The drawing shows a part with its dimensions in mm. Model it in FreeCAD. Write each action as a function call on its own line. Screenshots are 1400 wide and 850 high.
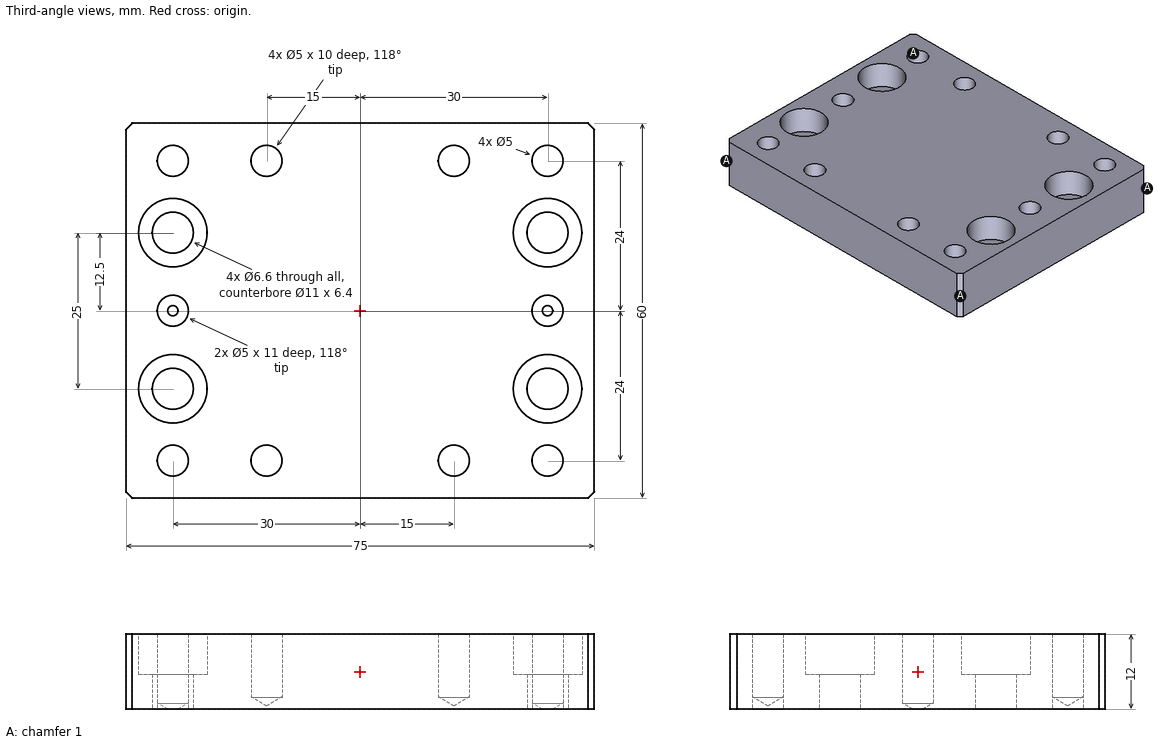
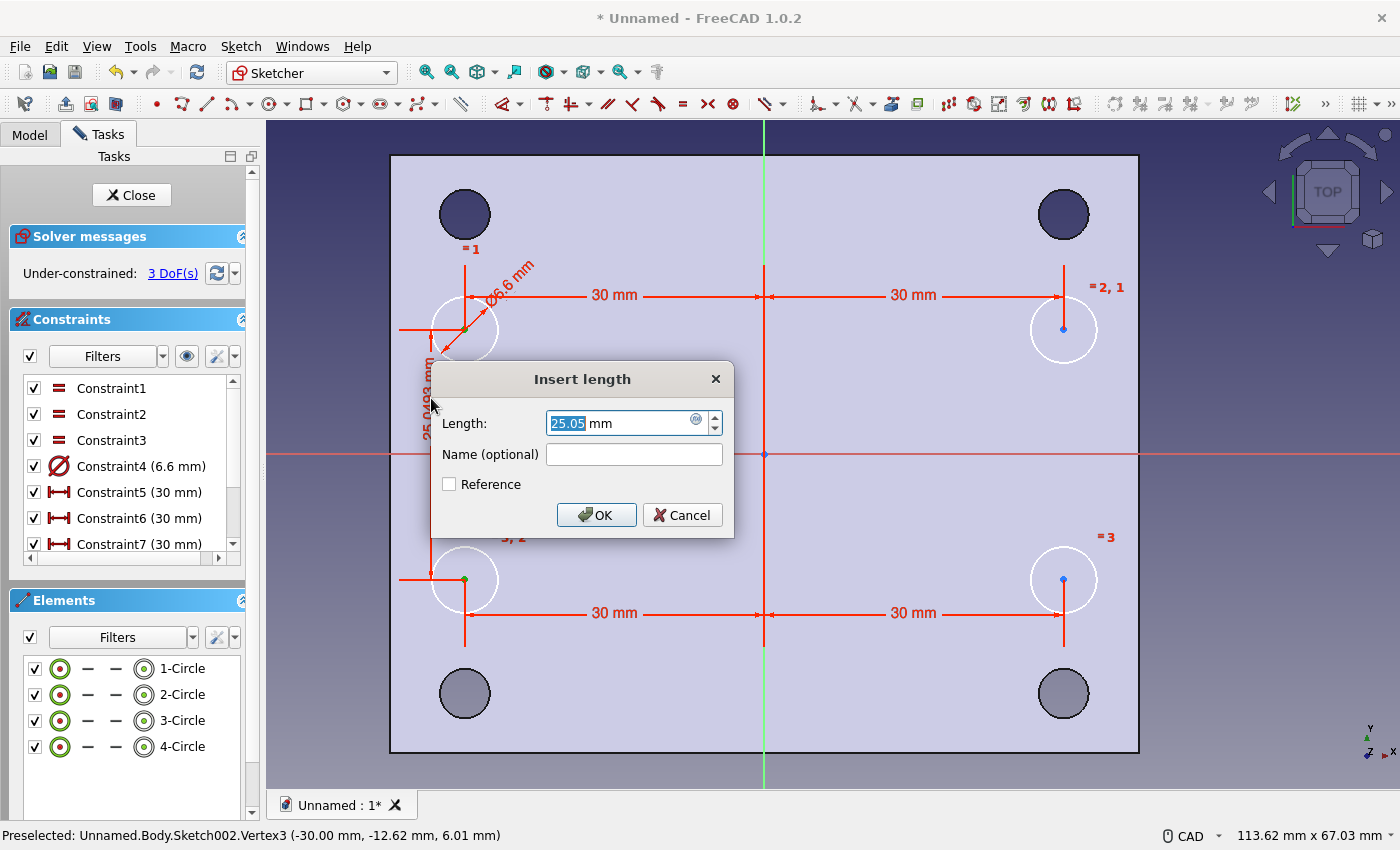
text(25)
key(Return)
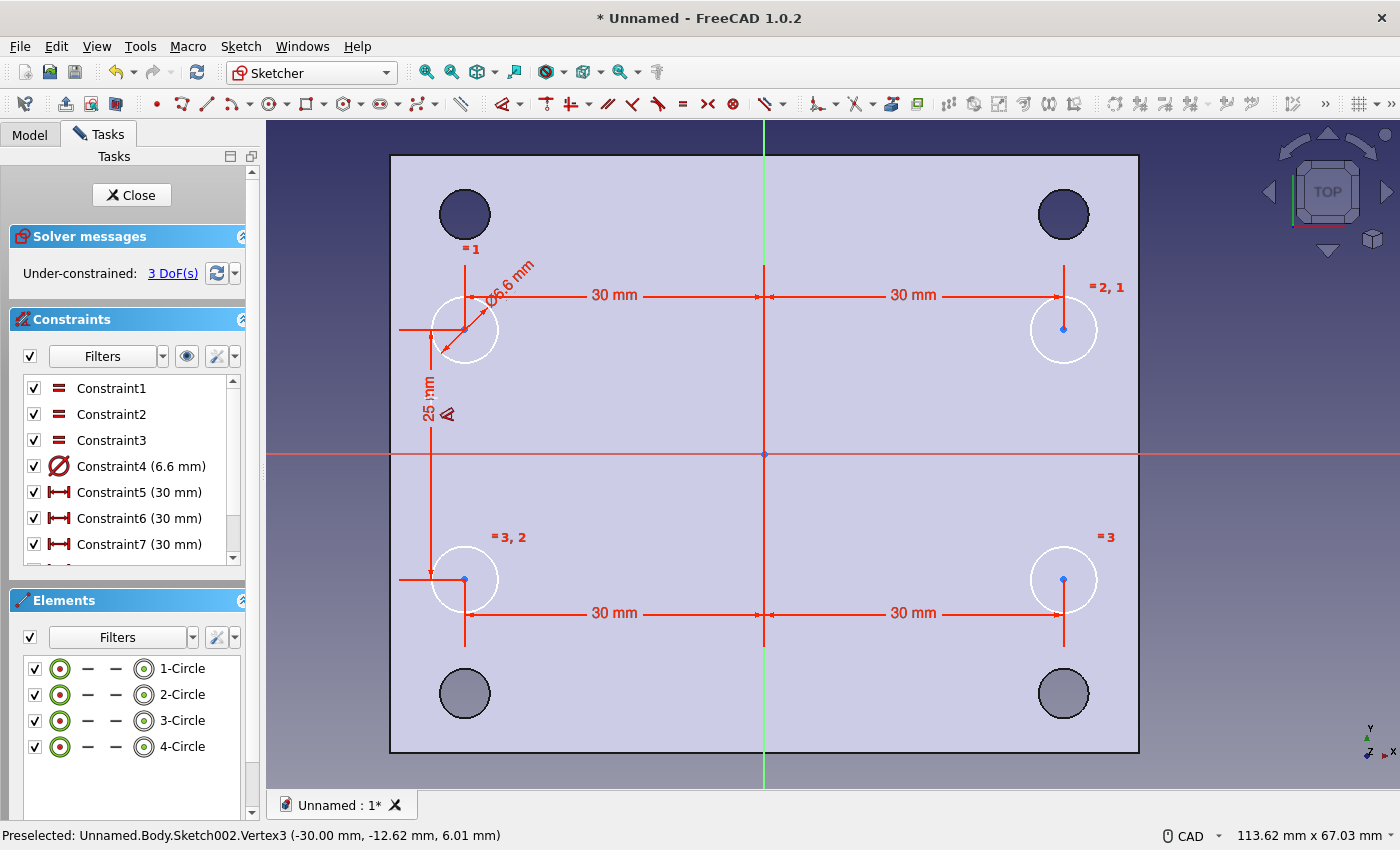
click(1064, 330)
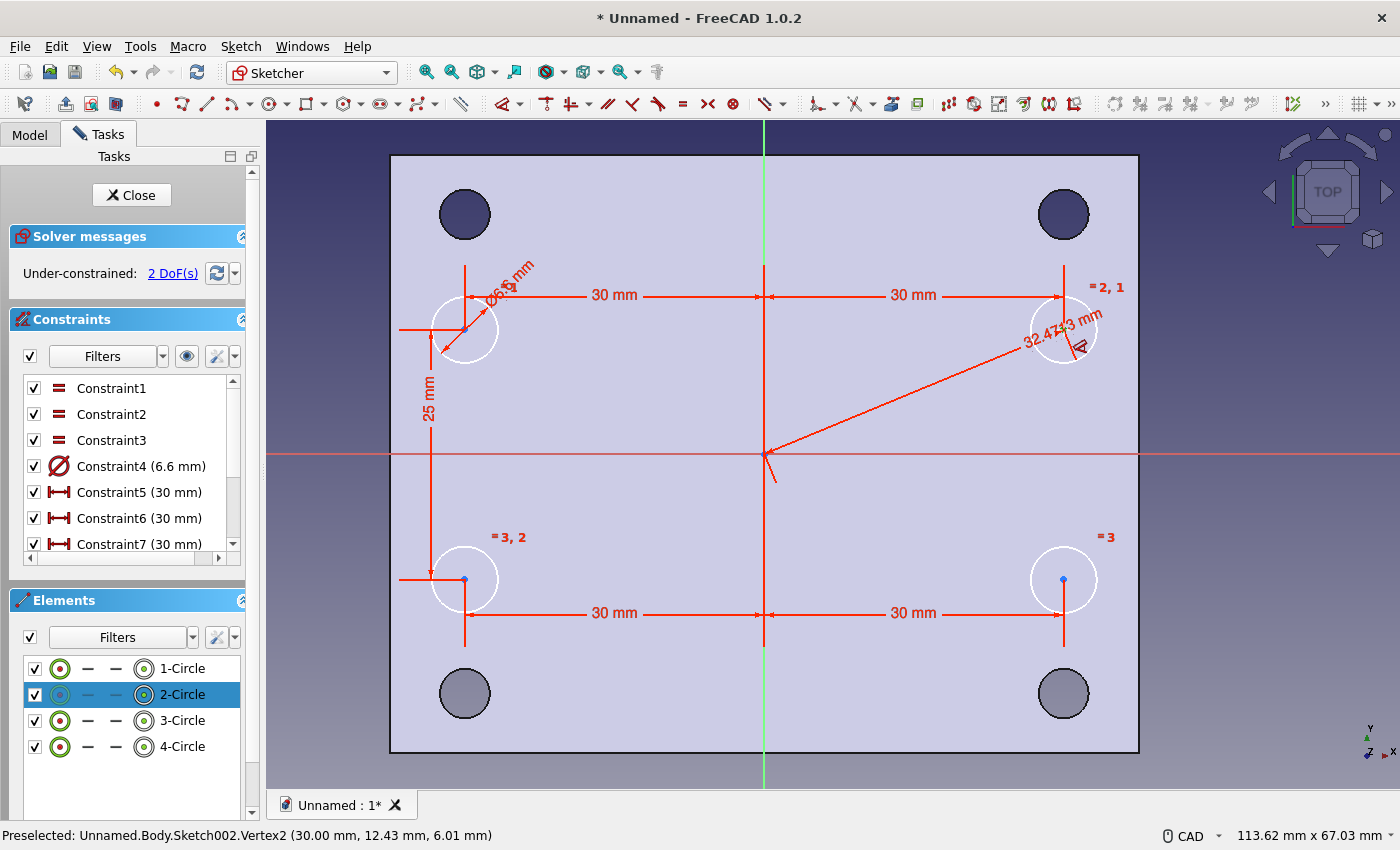
click(465, 580)
click(431, 512)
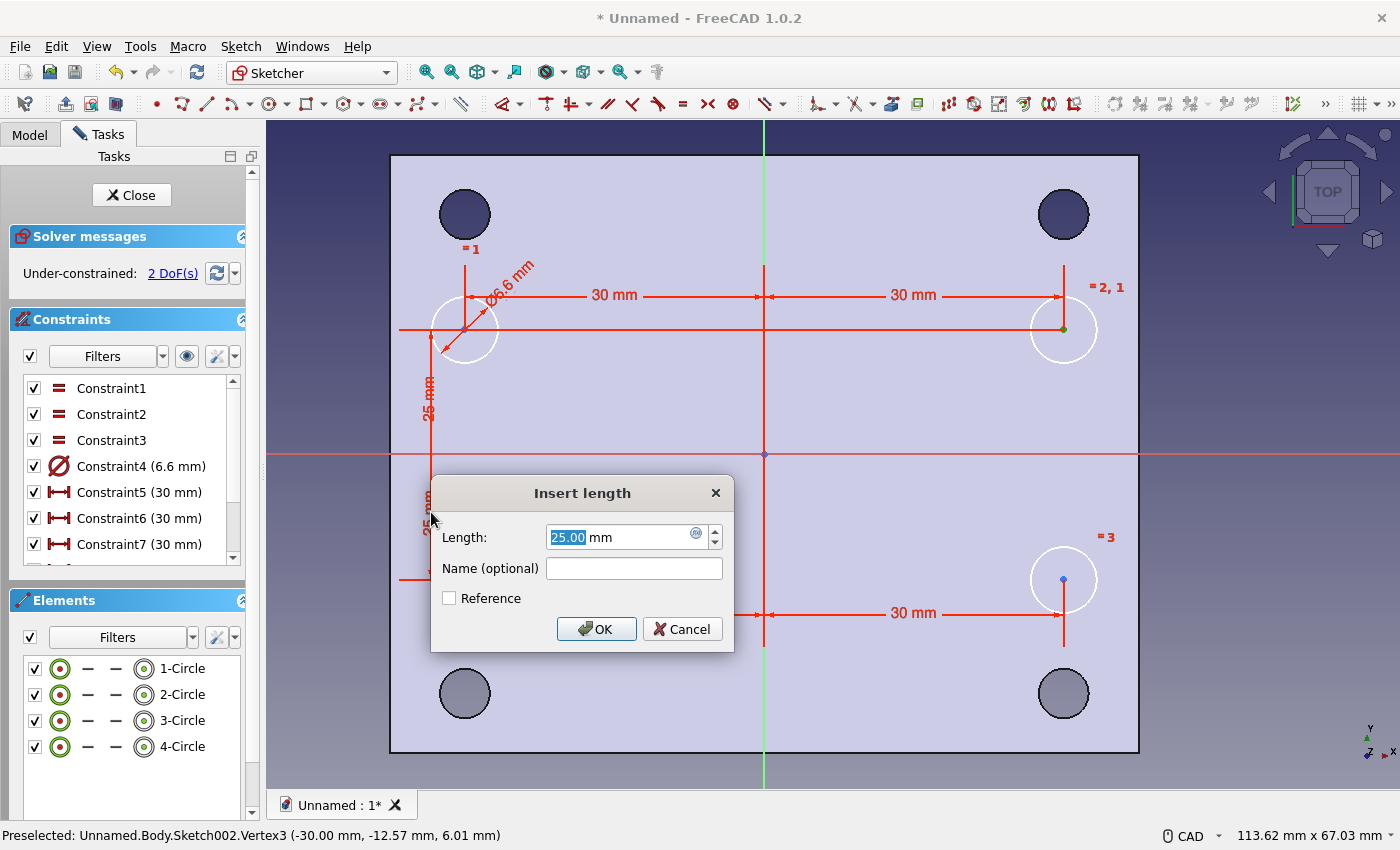
text(25)
key(Return)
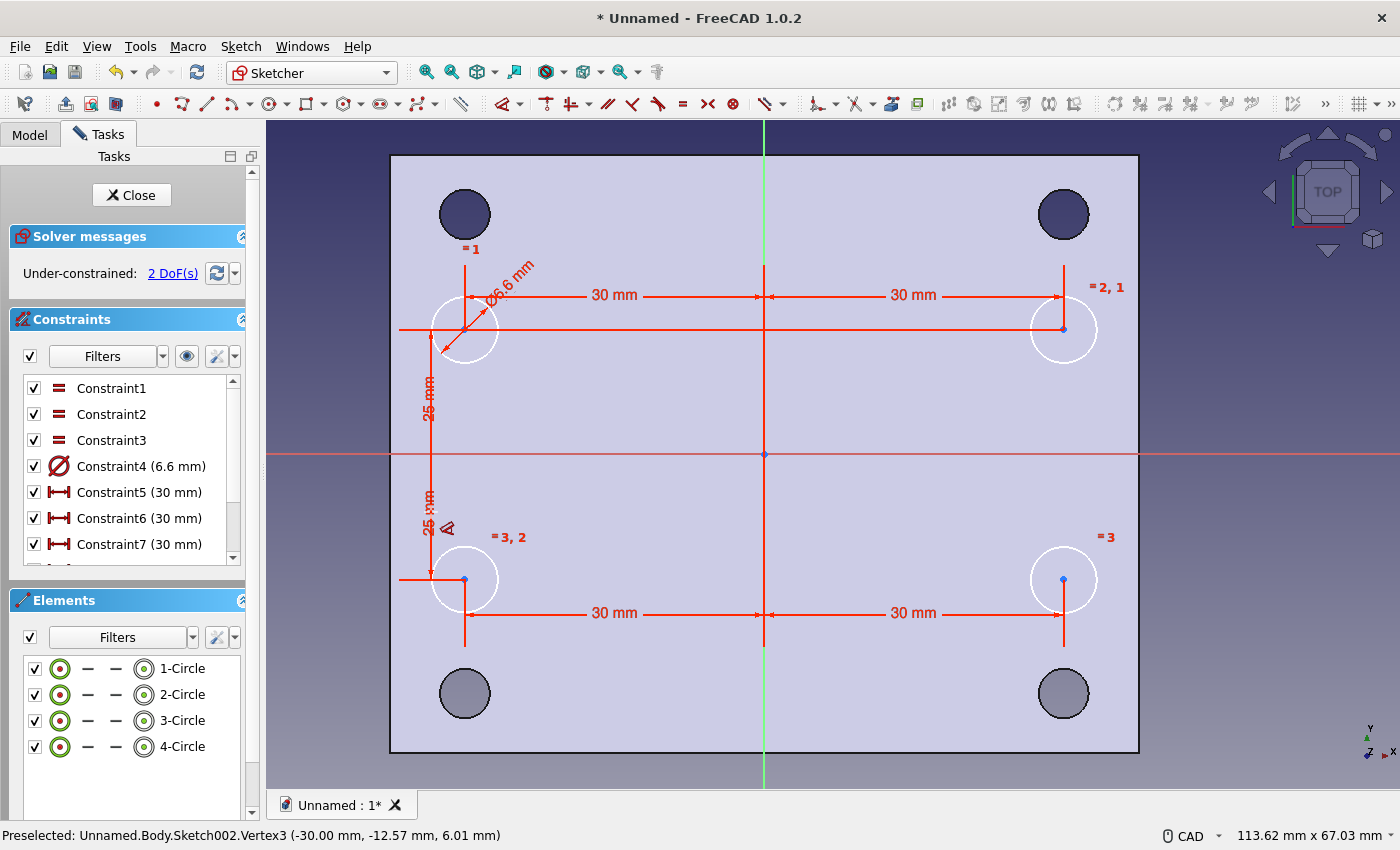
click(1064, 330)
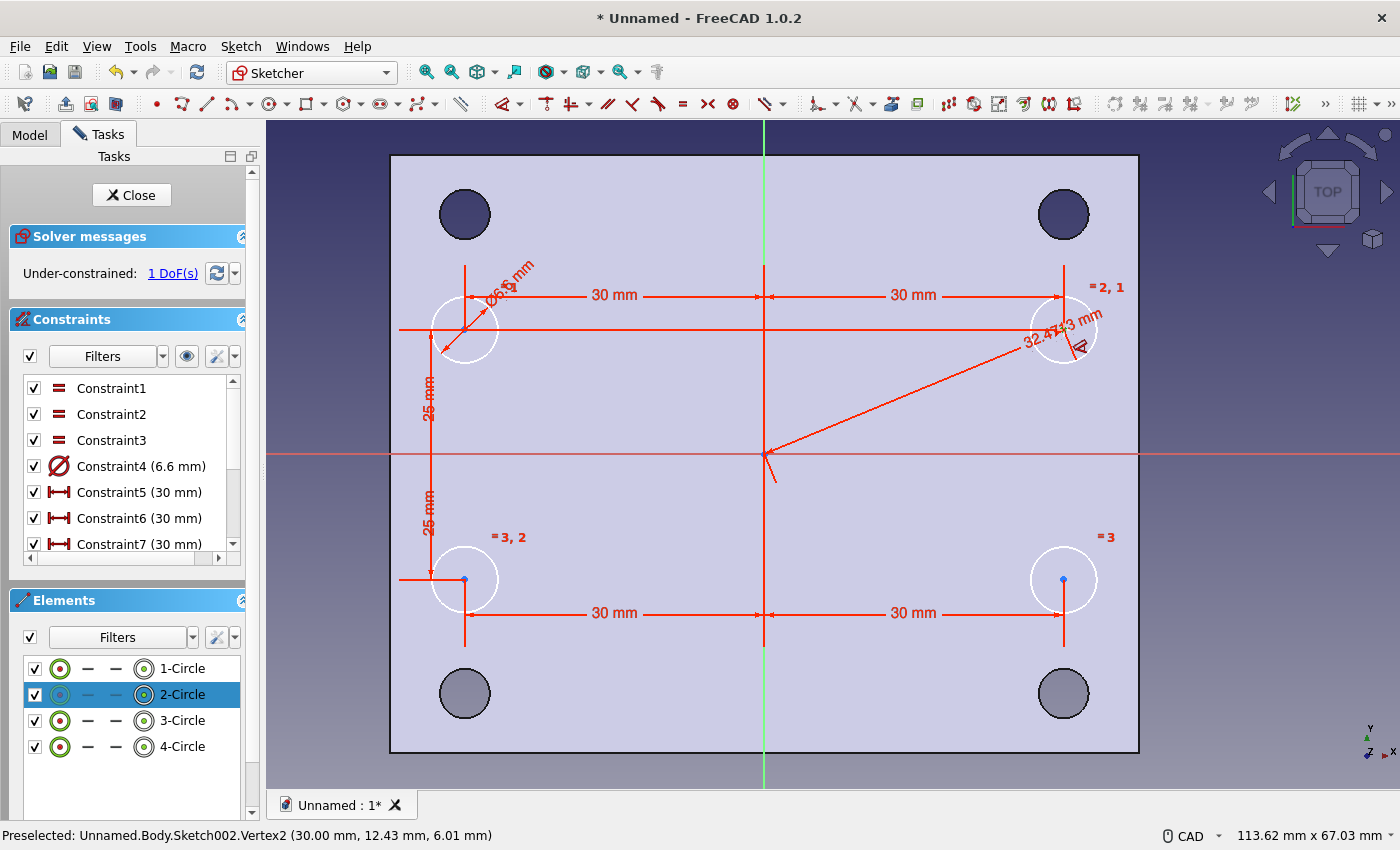
click(1064, 580)
click(1098, 398)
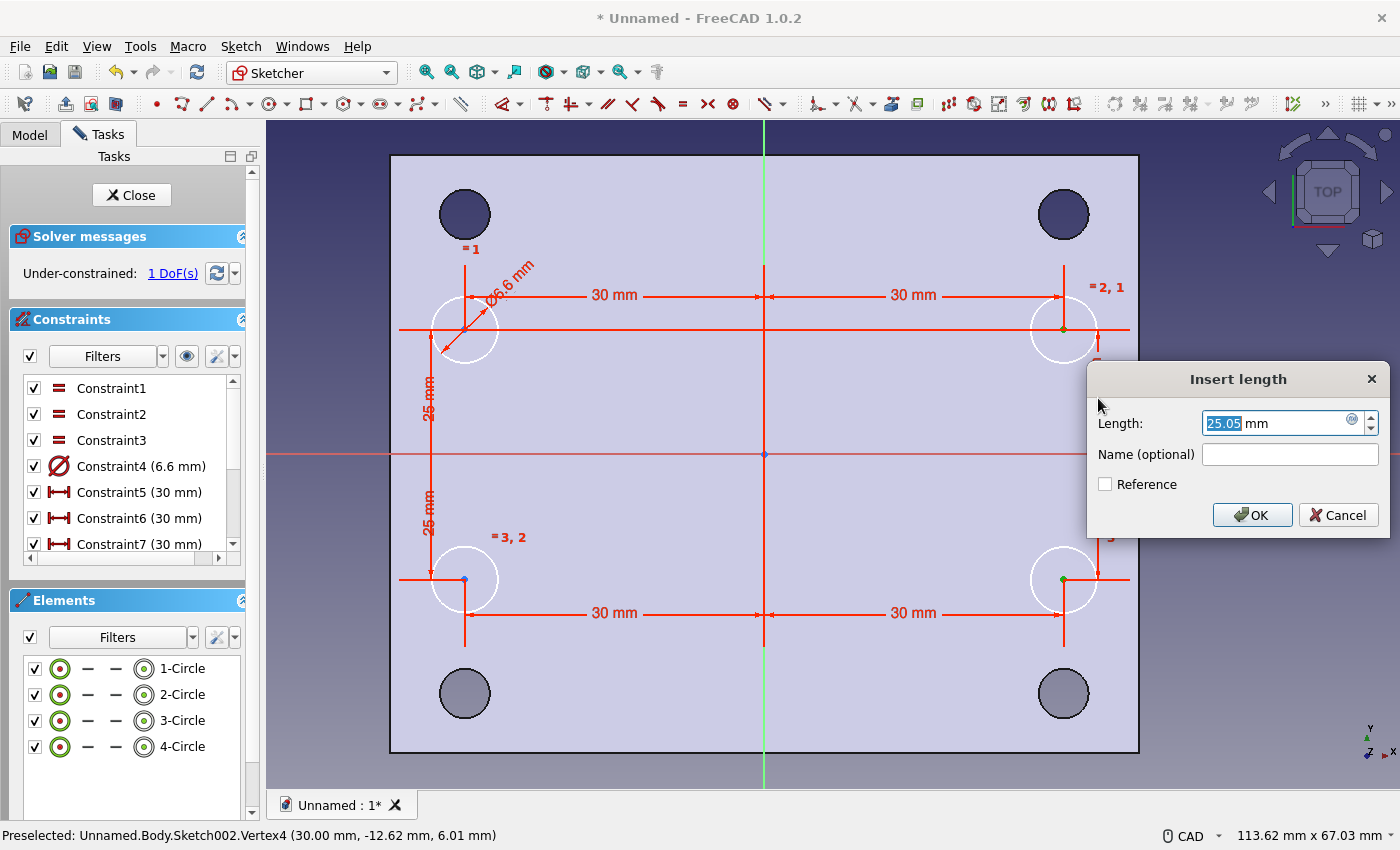
text(25)
key(Return)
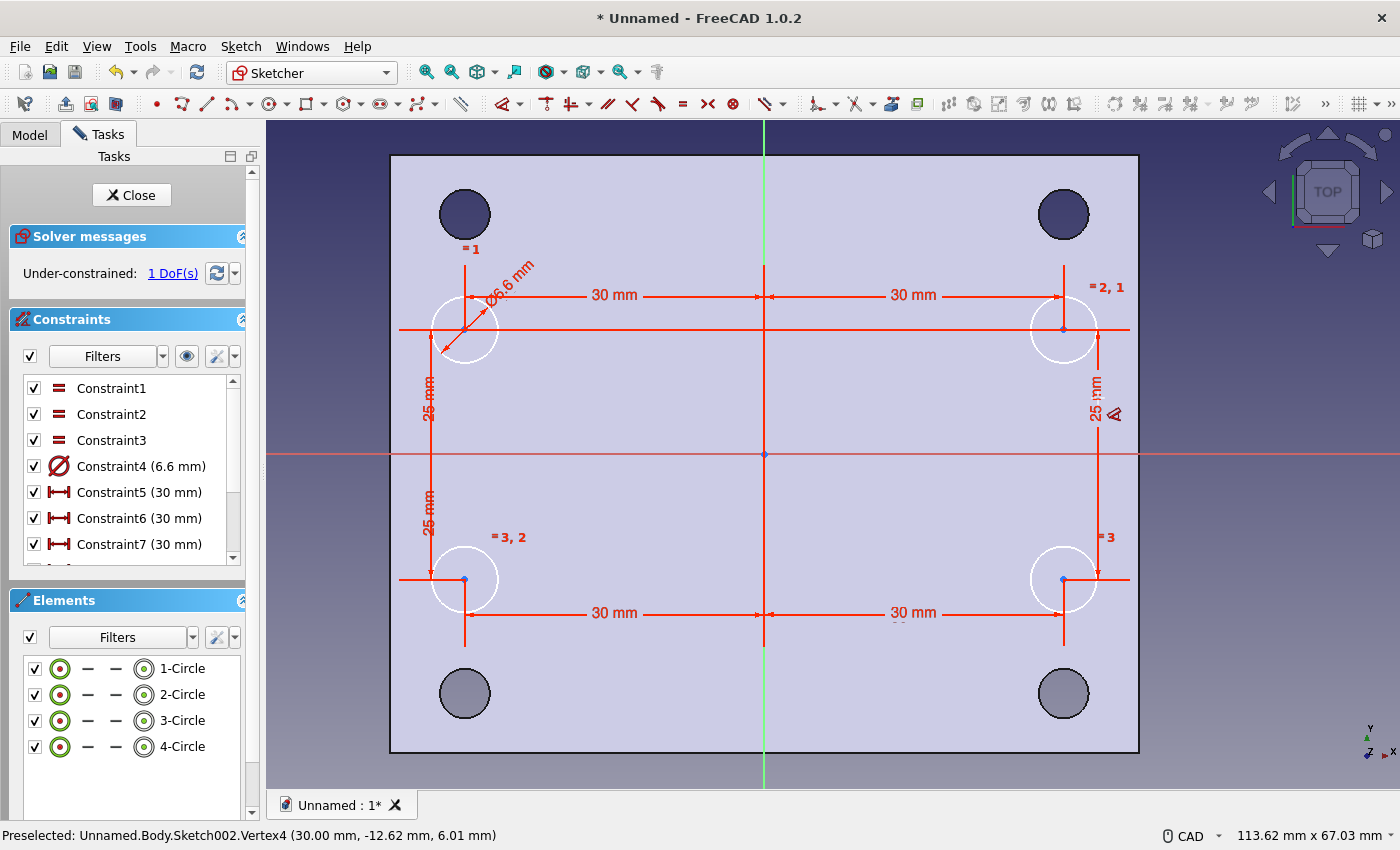
click(465, 330)
click(431, 363)